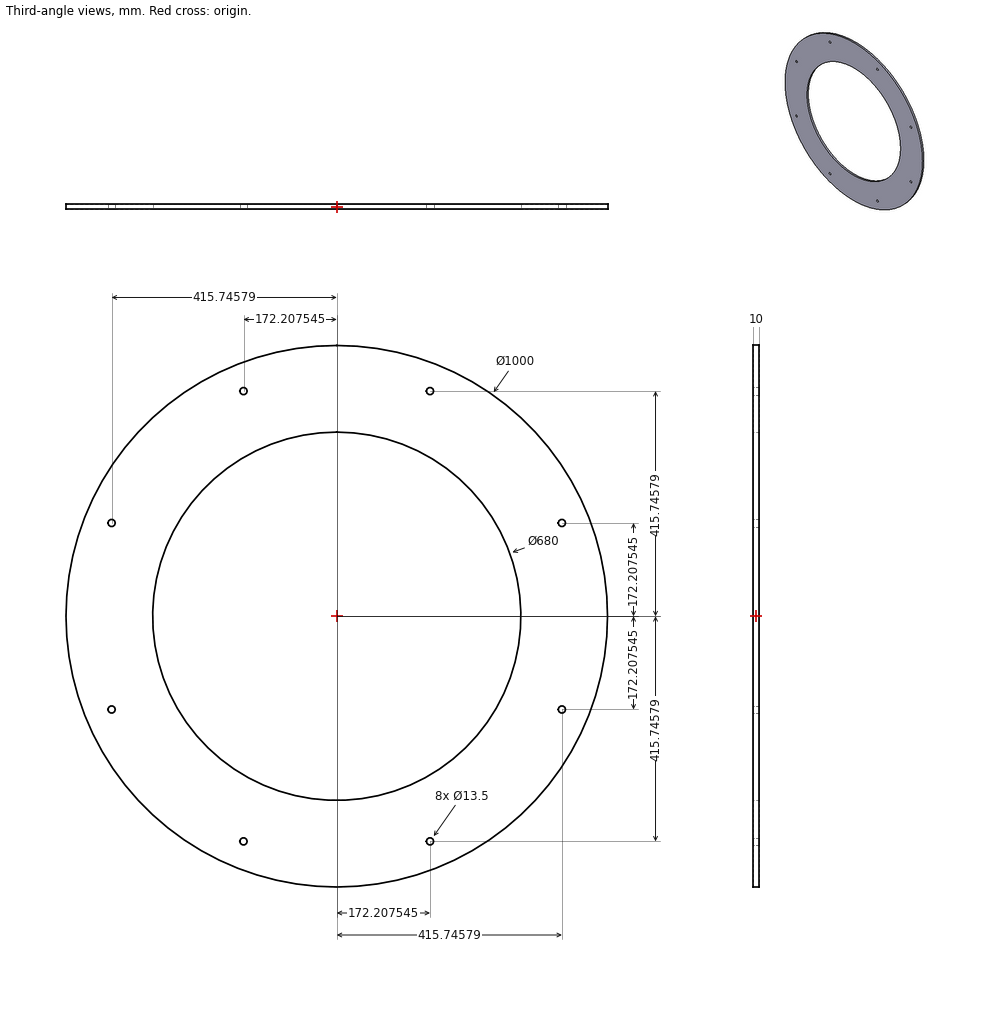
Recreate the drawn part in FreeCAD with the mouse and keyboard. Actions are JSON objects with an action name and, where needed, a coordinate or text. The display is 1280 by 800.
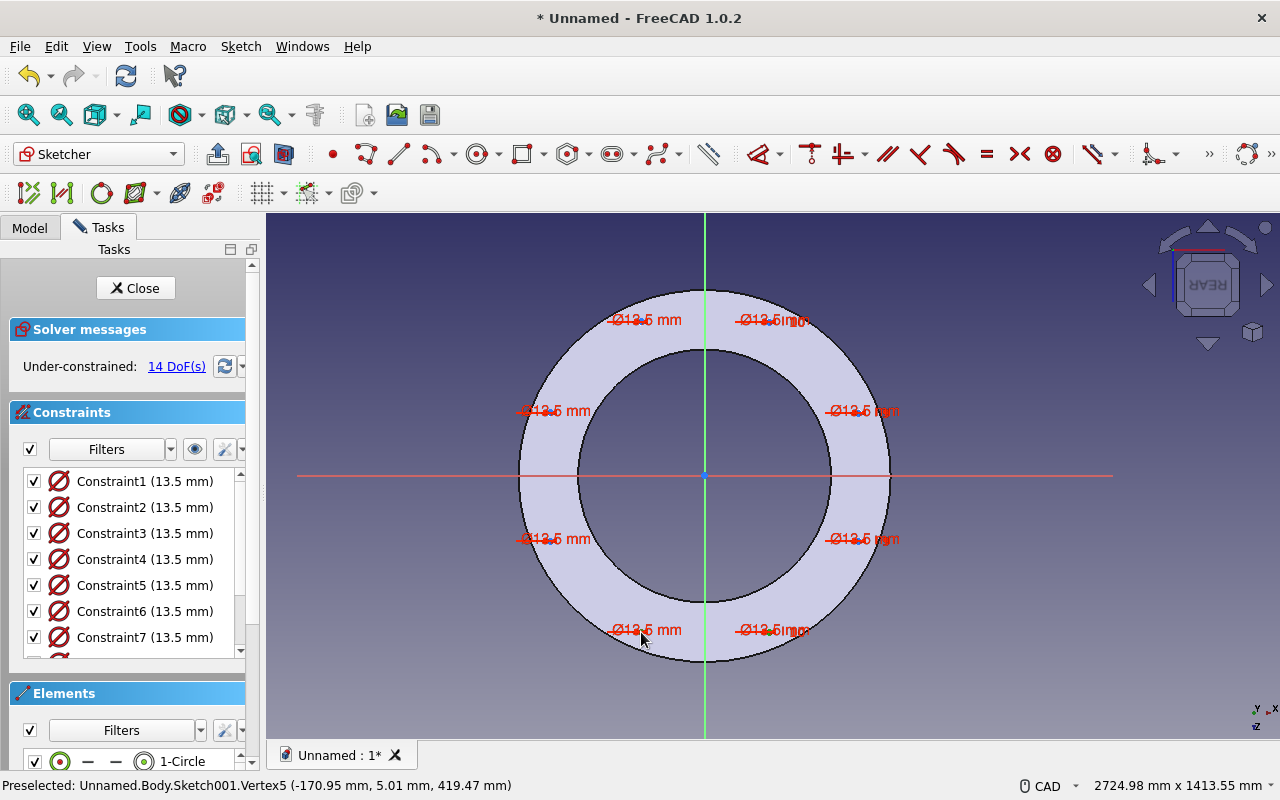
{"action": "key", "text": "h"}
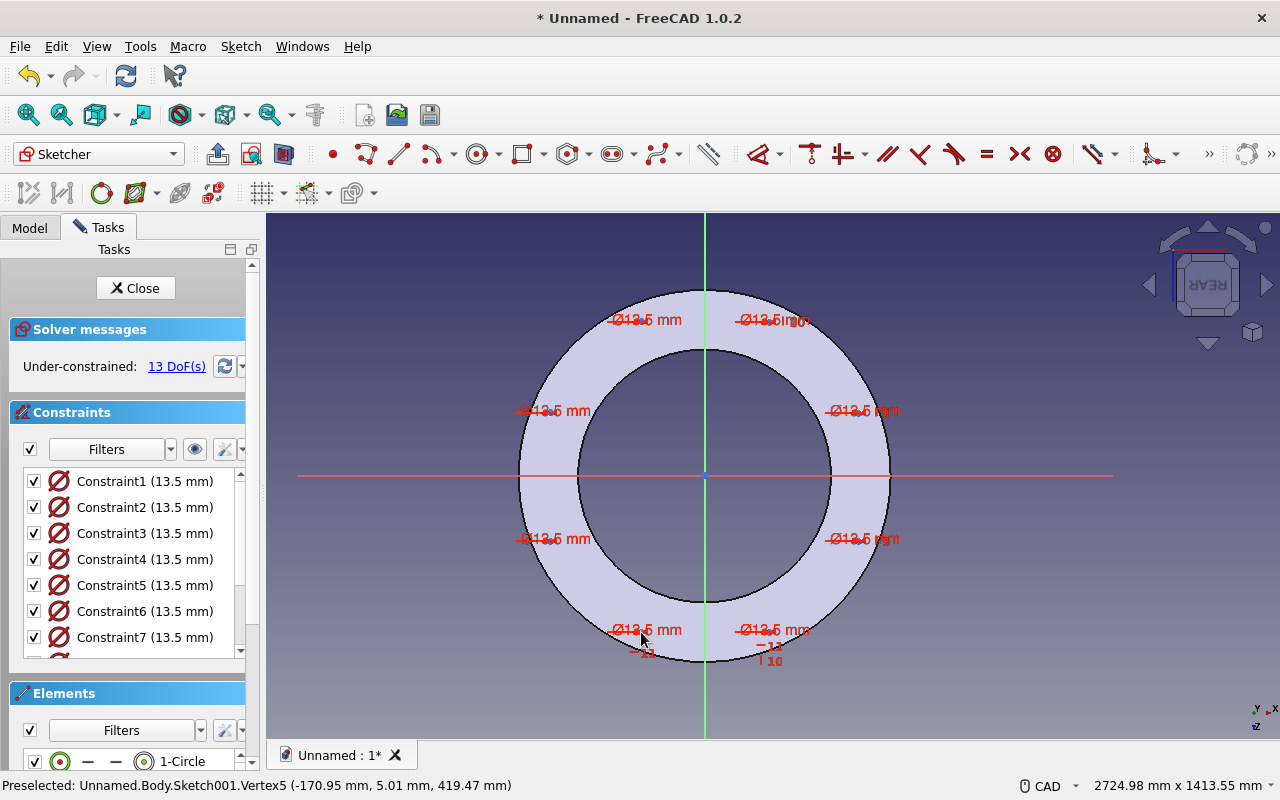
{"action": "left_click", "coordinate": [859, 541]}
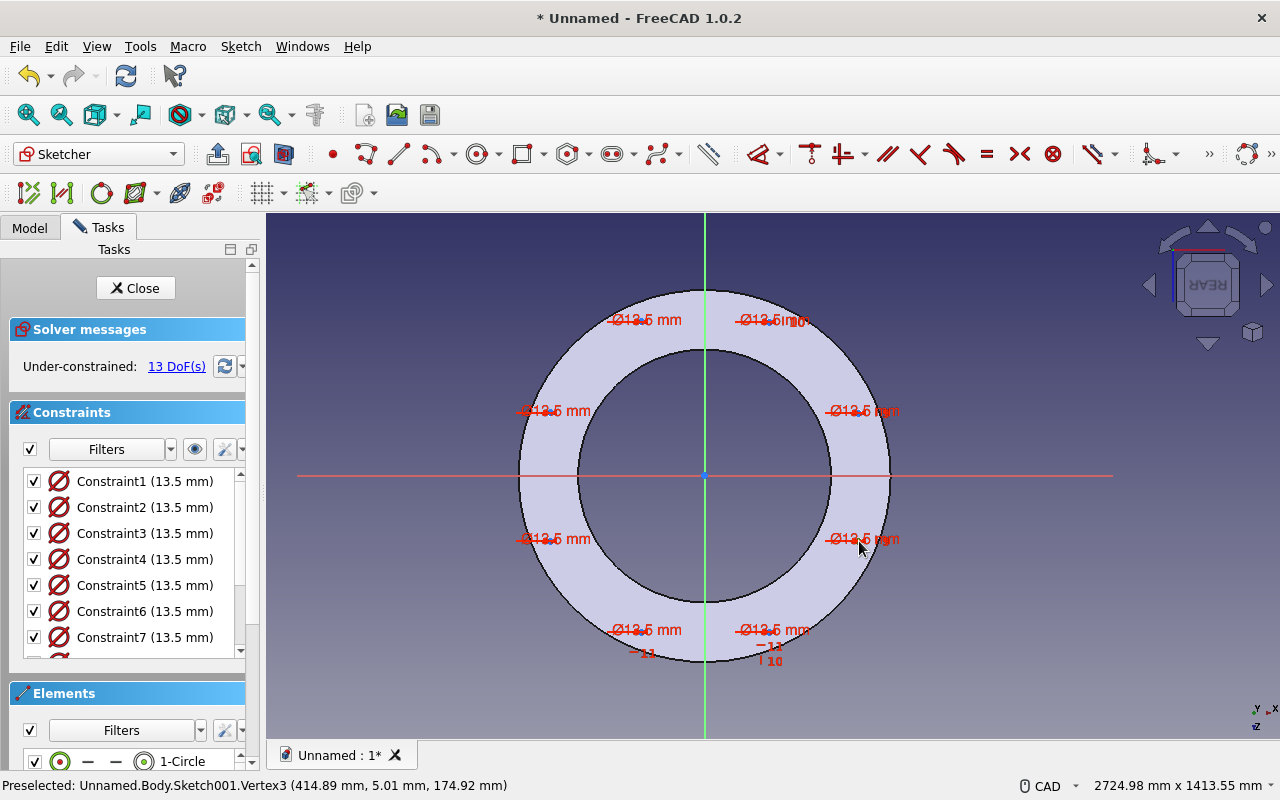
{"action": "left_click", "coordinate": [550, 541]}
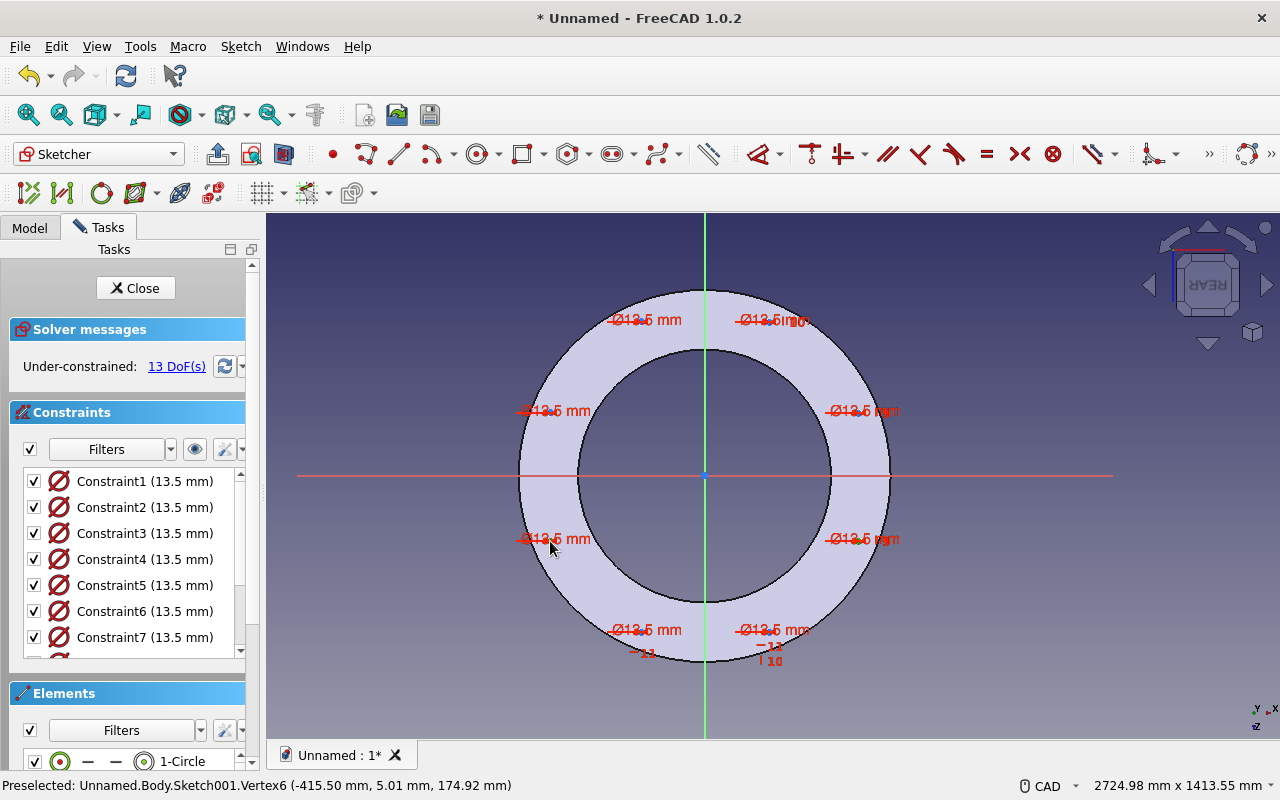
{"action": "key", "text": "h"}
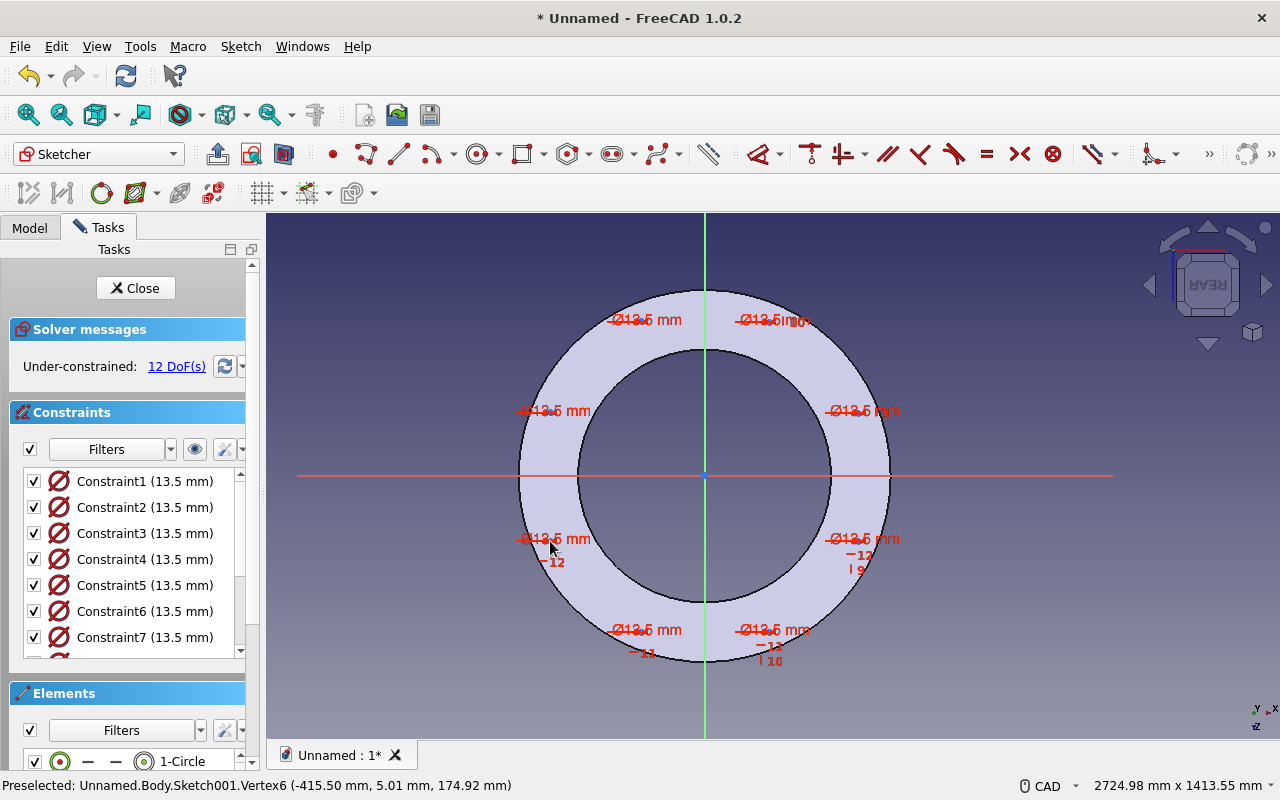
{"action": "left_click", "coordinate": [550, 541]}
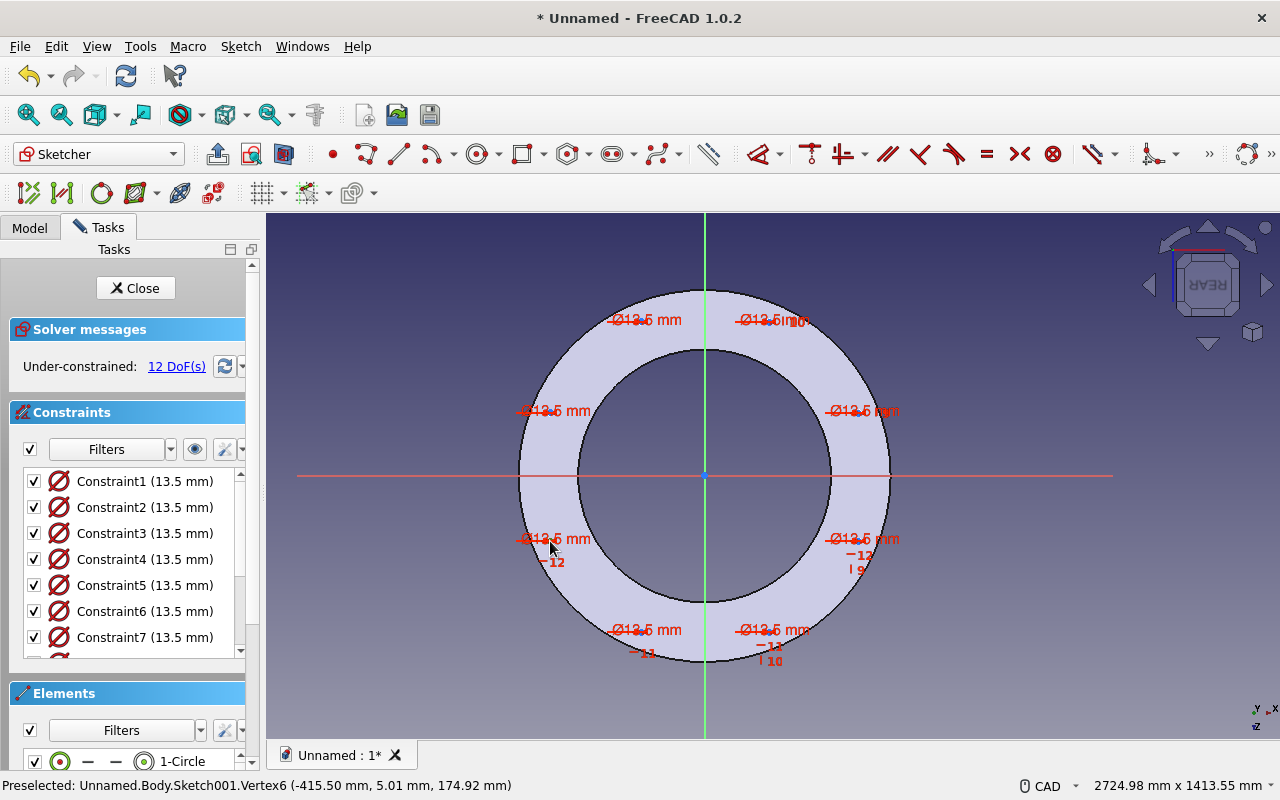
{"action": "left_click", "coordinate": [550, 413]}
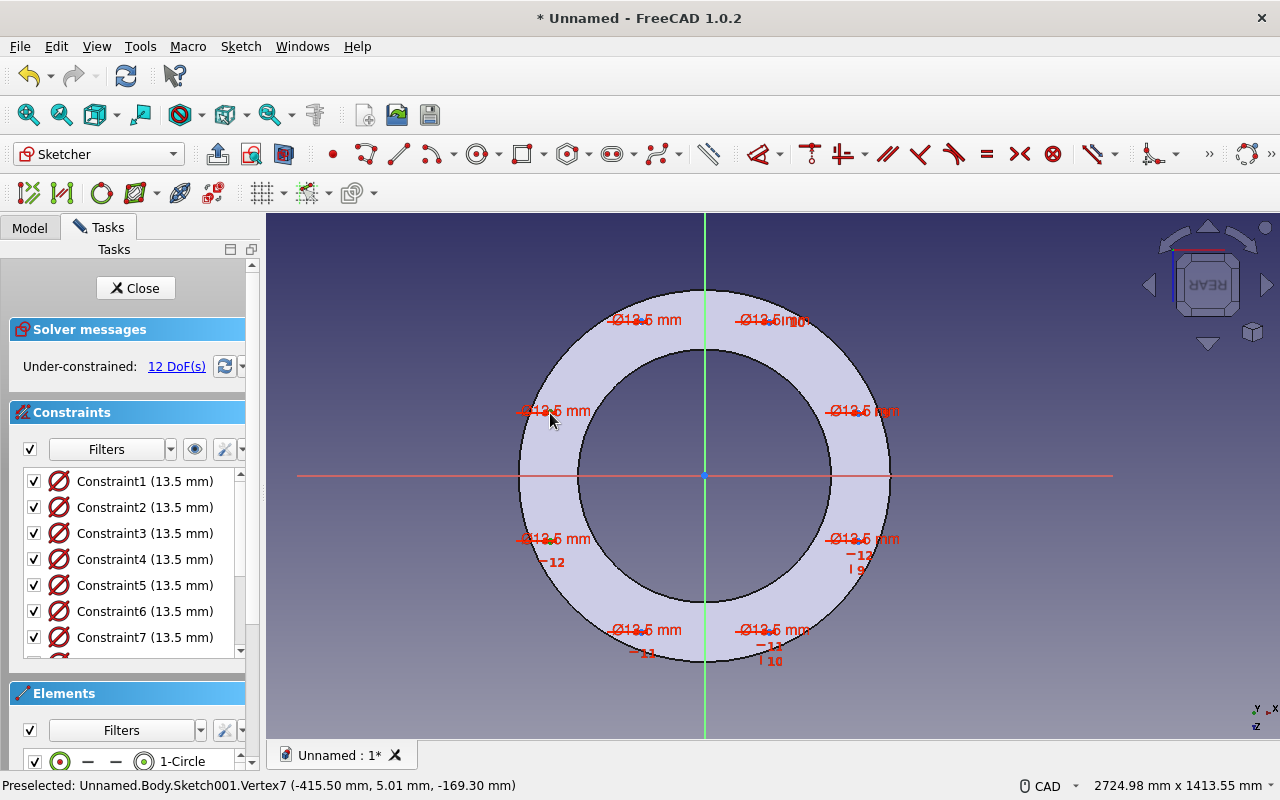
{"action": "key", "text": "v"}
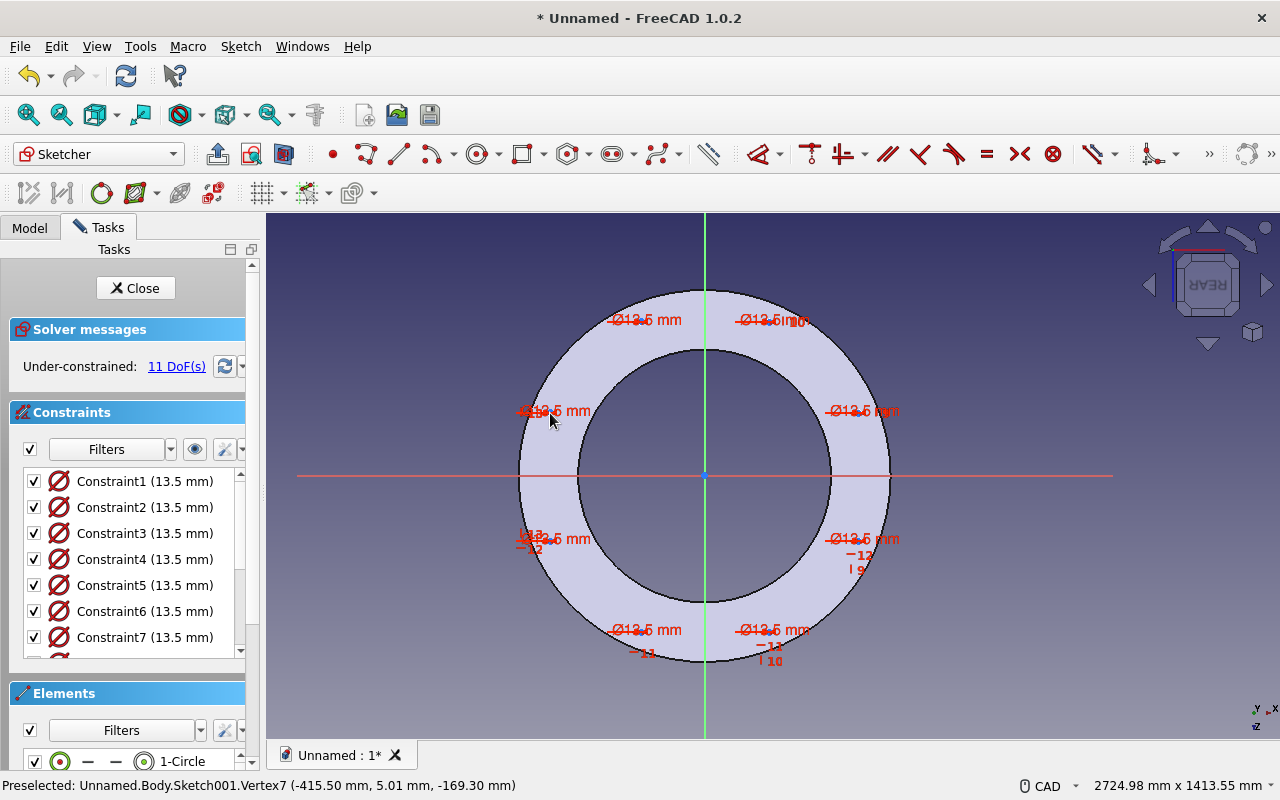
{"action": "left_click", "coordinate": [859, 413]}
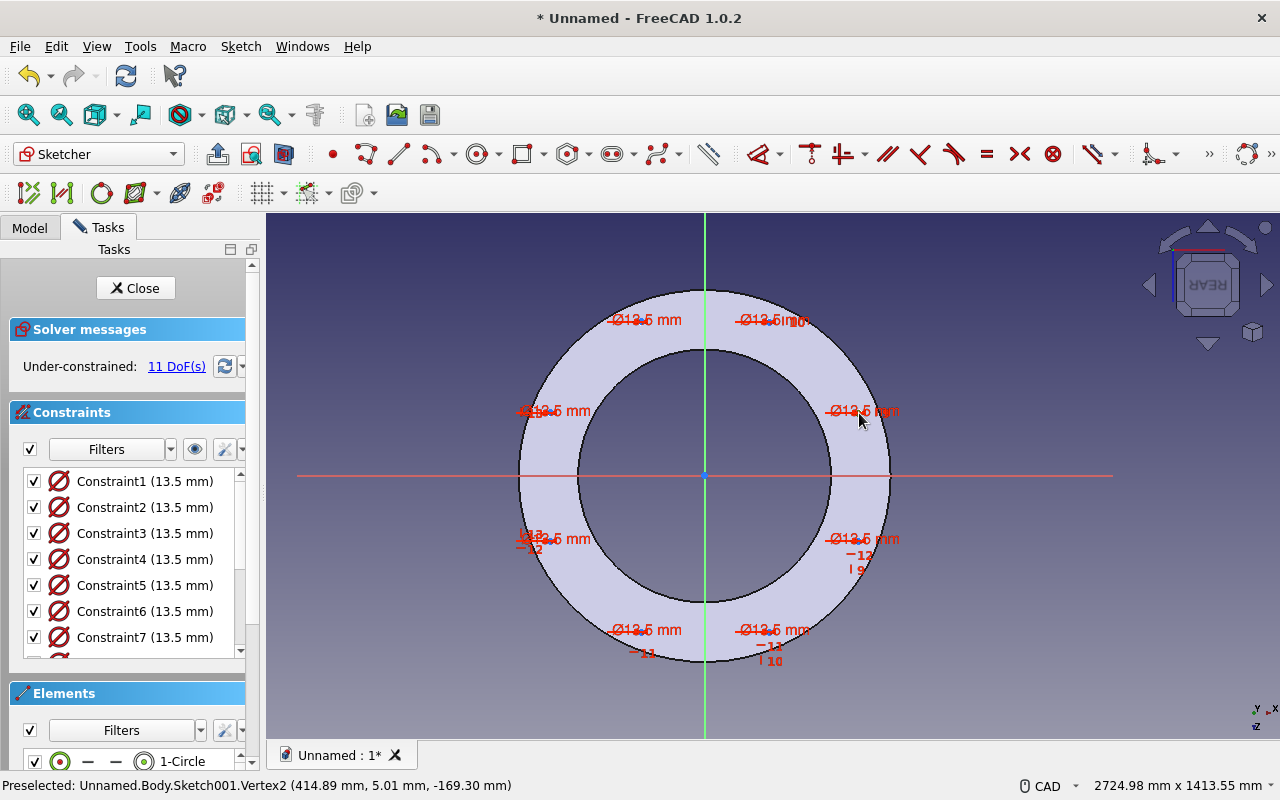
{"action": "left_click", "coordinate": [550, 413]}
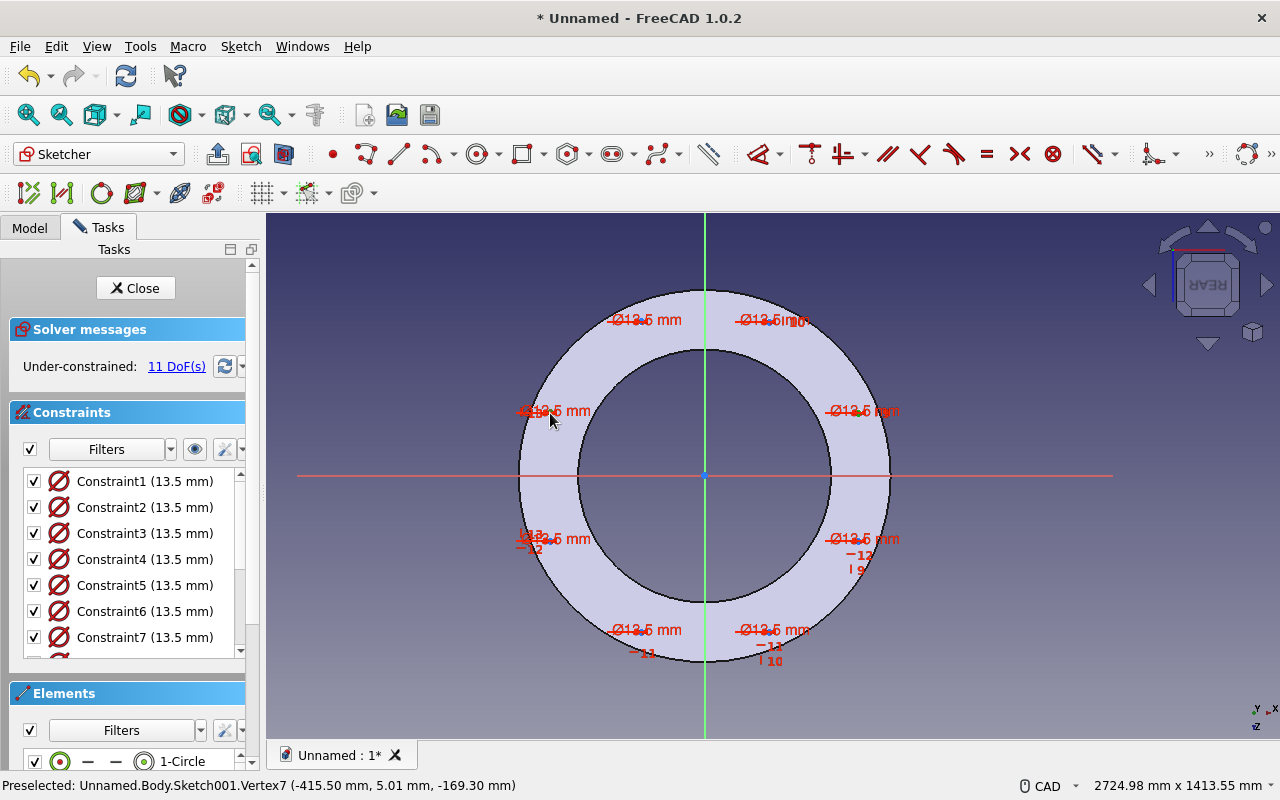
{"action": "left_click", "coordinate": [864, 154]}